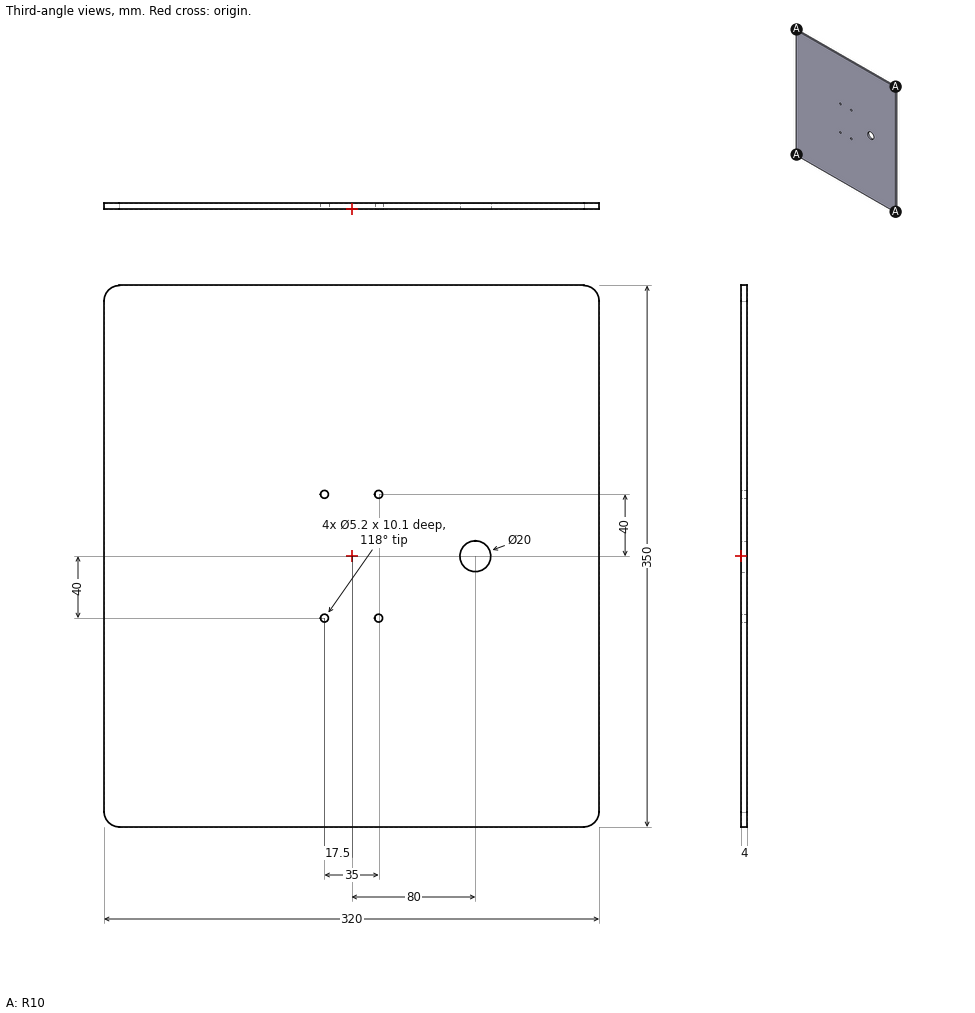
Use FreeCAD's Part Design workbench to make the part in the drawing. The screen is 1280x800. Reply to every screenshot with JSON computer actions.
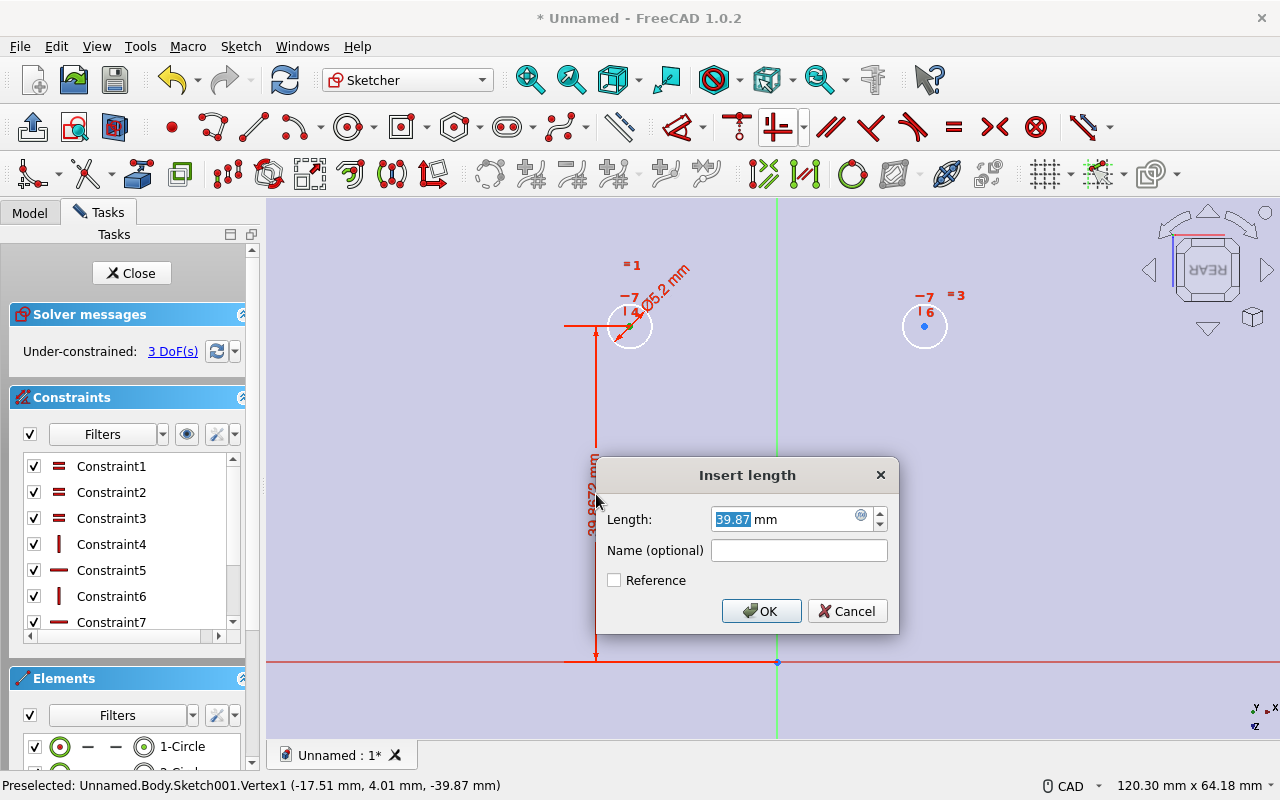
{"action": "type", "text": "40"}
{"action": "key", "text": "Return"}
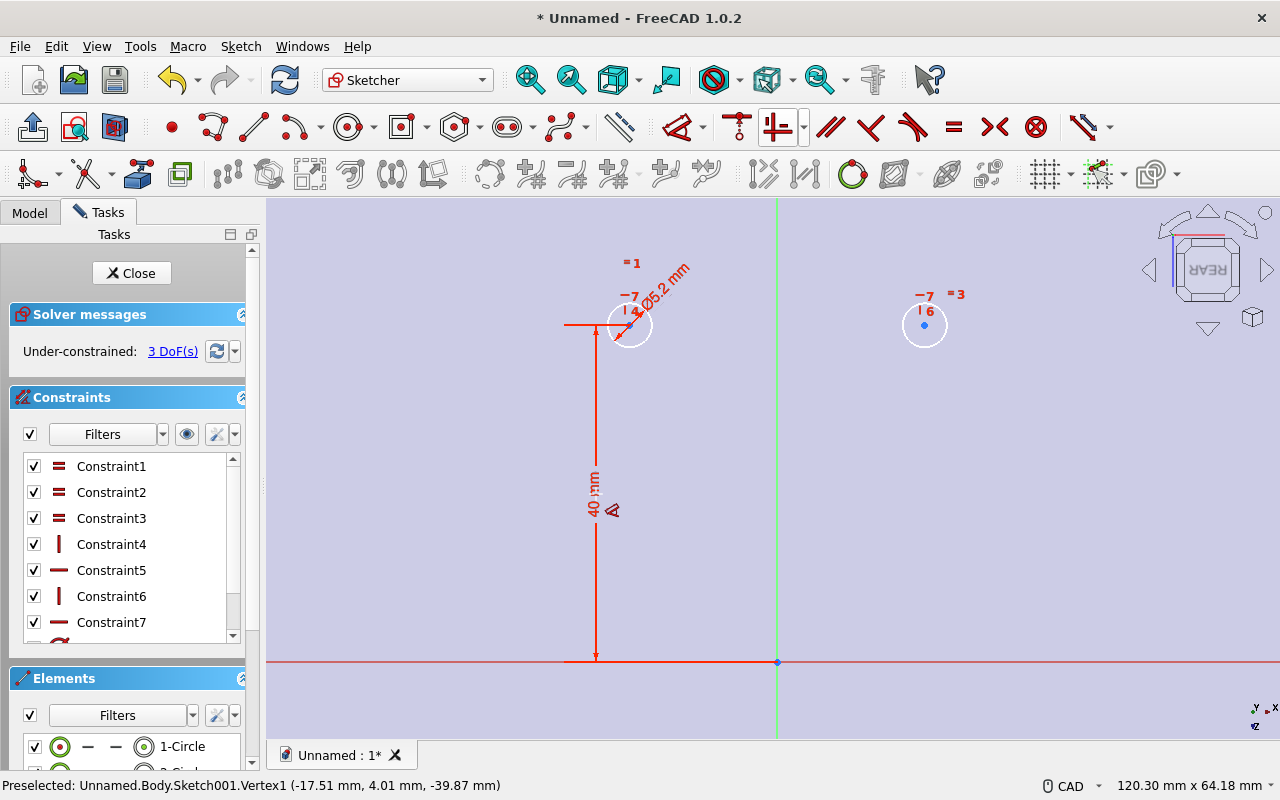
{"action": "scroll", "coordinate": [645, 310], "scroll_direction": "down", "scroll_amount": 4}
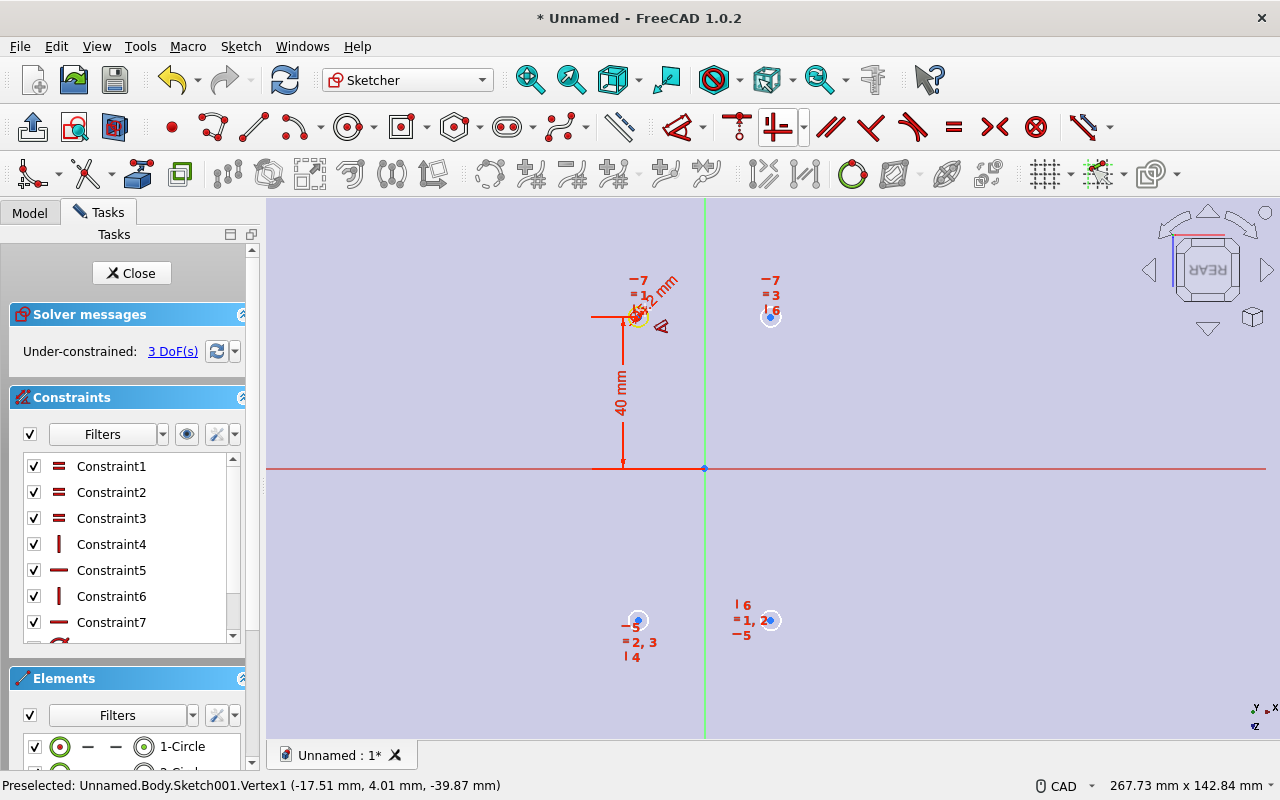
{"action": "left_click", "coordinate": [771, 620]}
{"action": "left_click", "coordinate": [805, 544]}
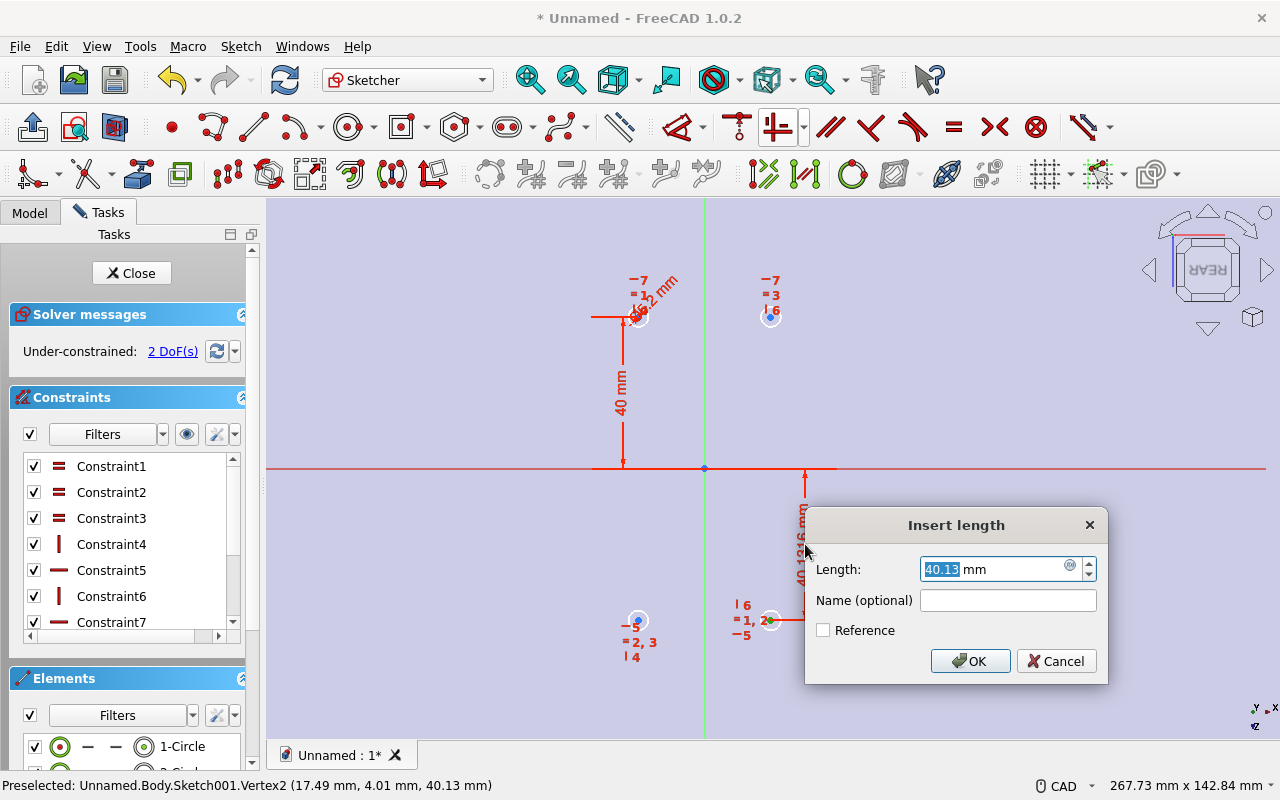
{"action": "type", "text": "40"}
{"action": "key", "text": "Return"}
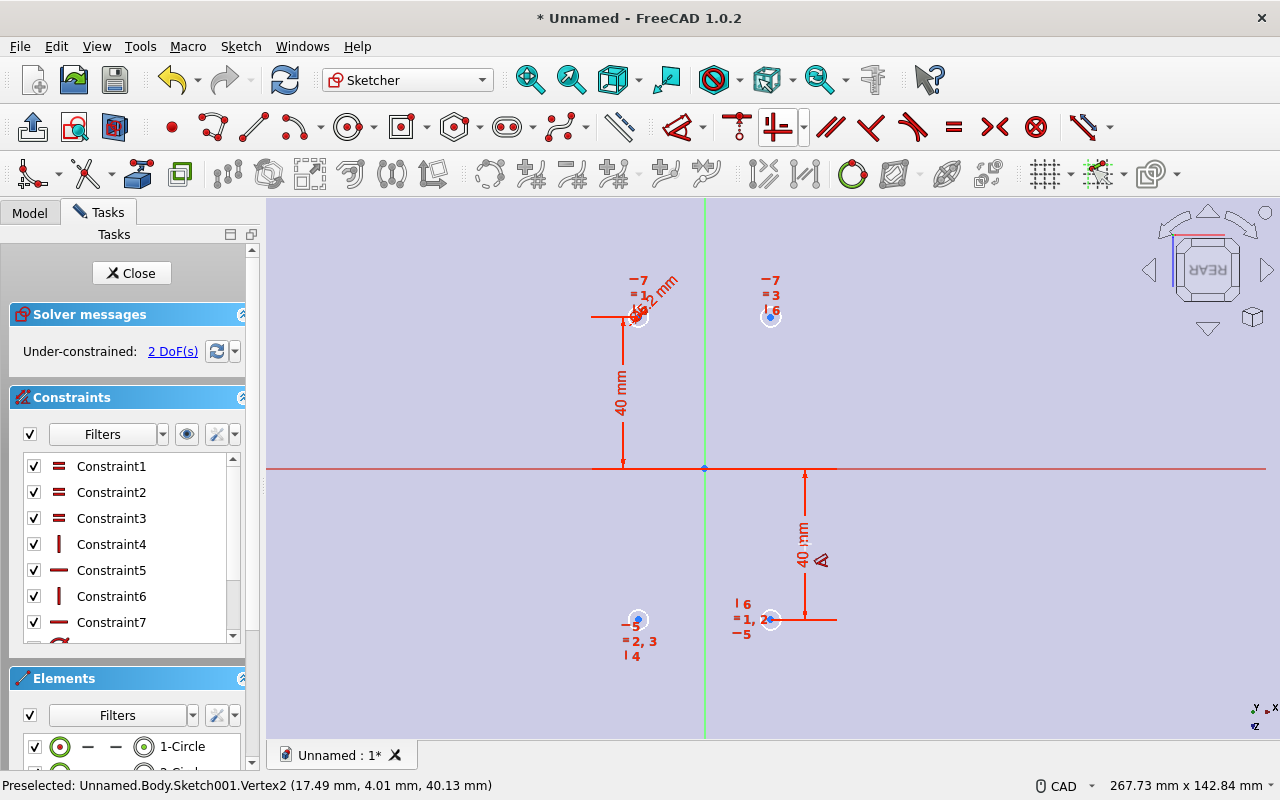
{"action": "left_click", "coordinate": [638, 317]}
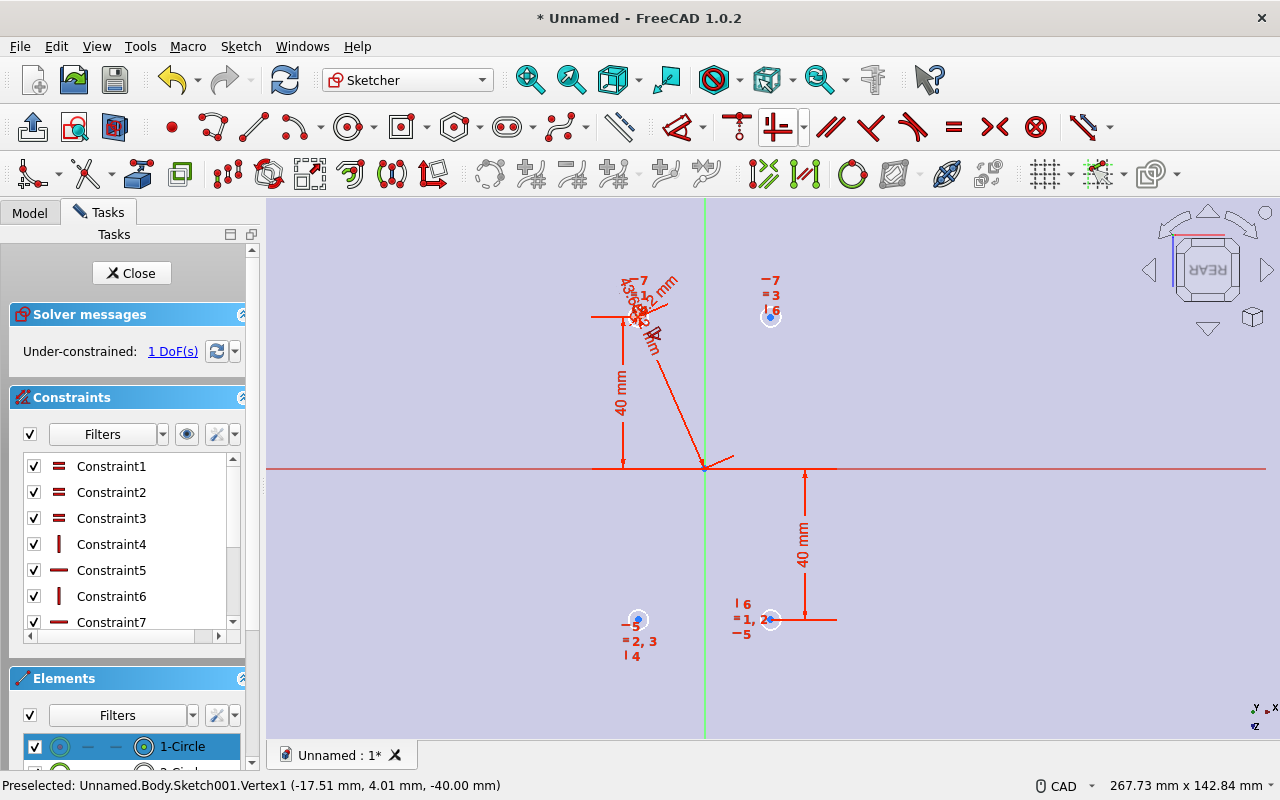
{"action": "left_click", "coordinate": [771, 620]}
{"action": "left_click", "coordinate": [735, 283]}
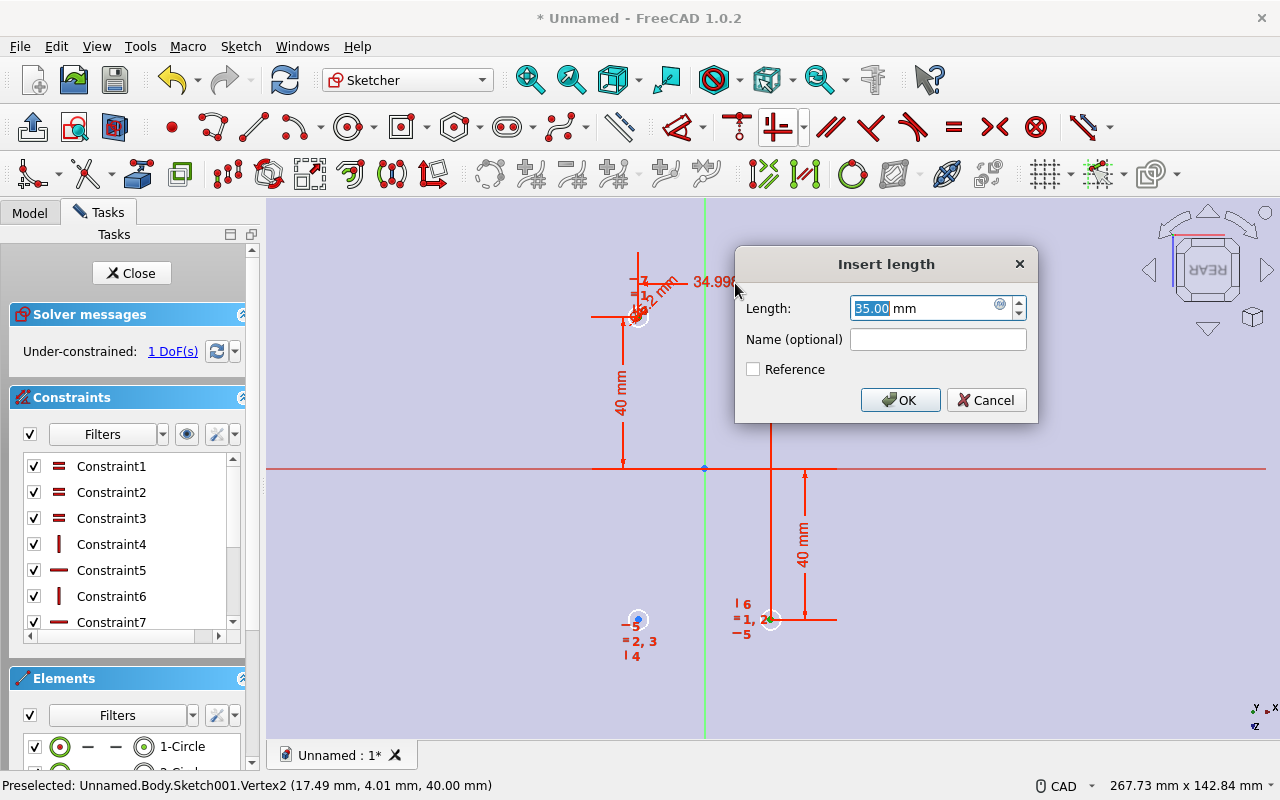
{"action": "type", "text": "35"}
{"action": "key", "text": "Return"}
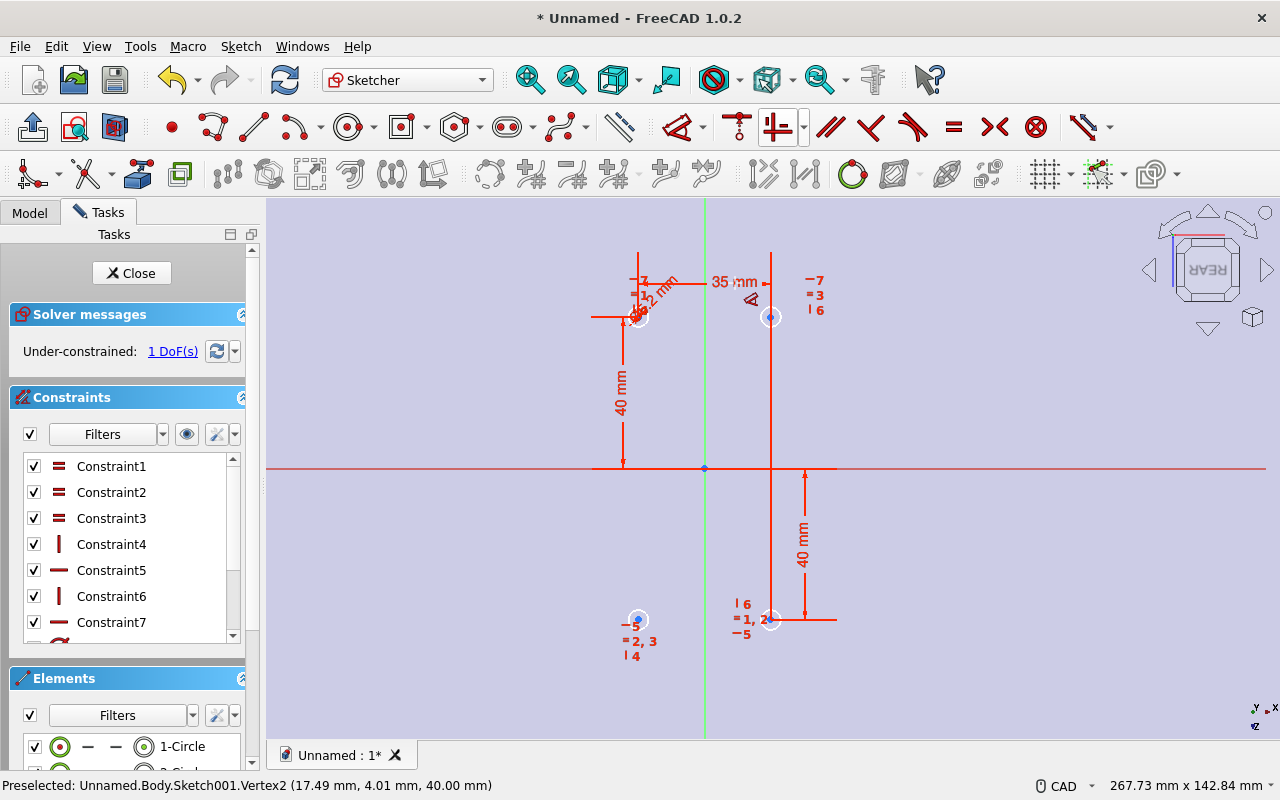
{"action": "left_click", "coordinate": [638, 317]}
{"action": "left_click", "coordinate": [672, 502]}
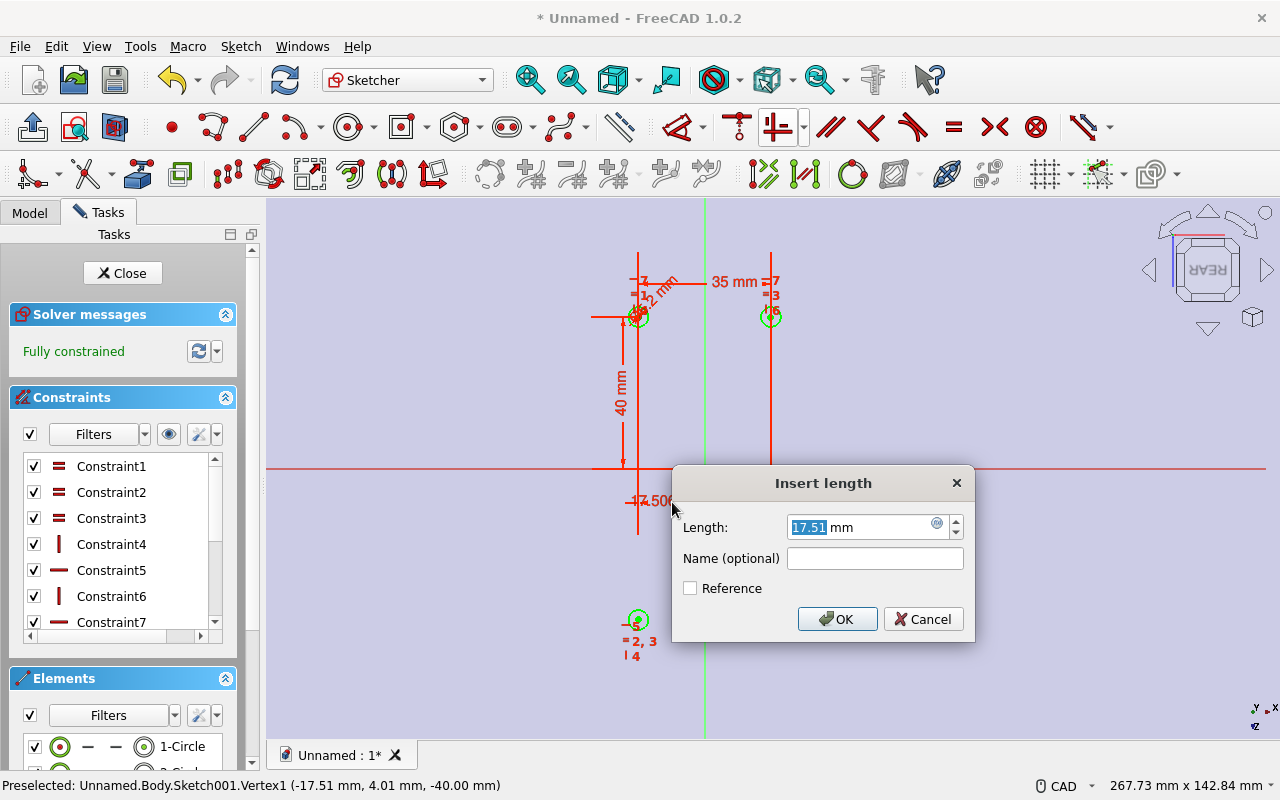
{"action": "type", "text": "17.5"}
{"action": "key", "text": "Return"}
{"action": "key", "text": "Escape"}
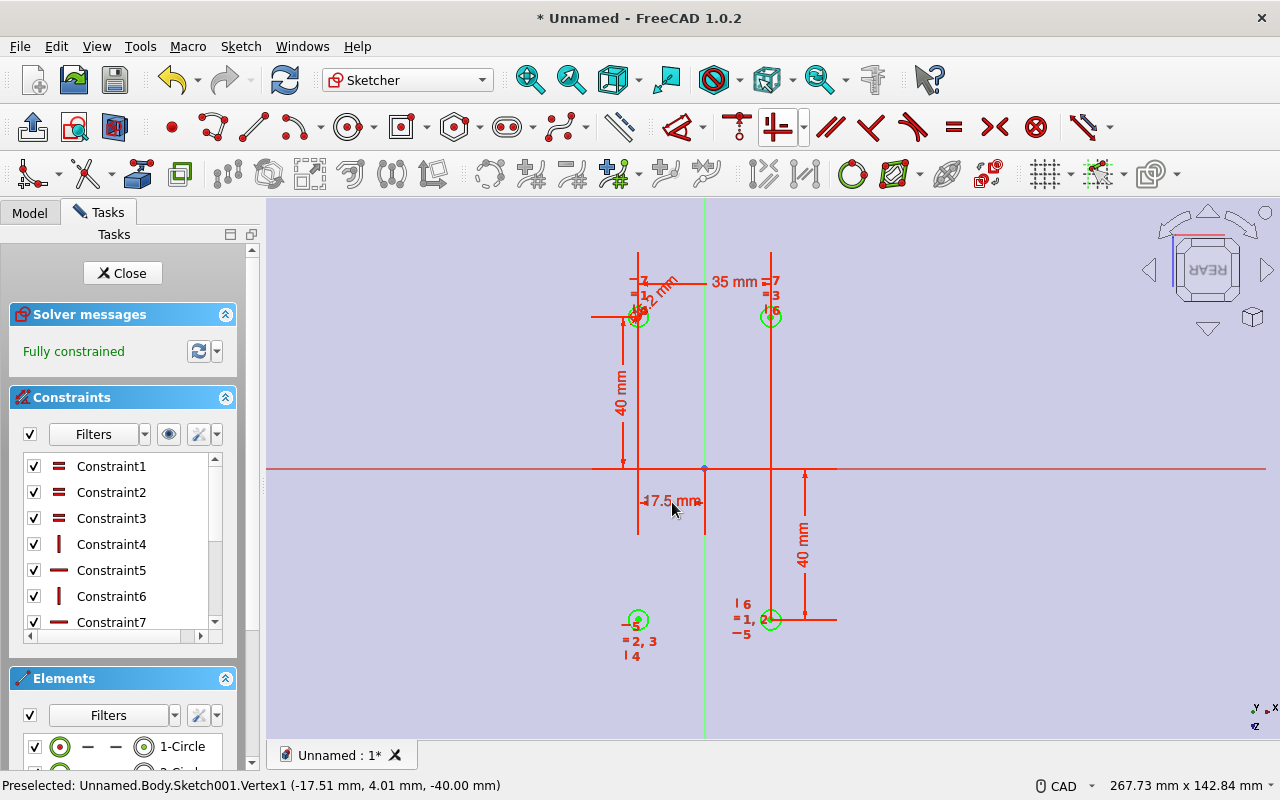
{"action": "left_click", "coordinate": [123, 273]}